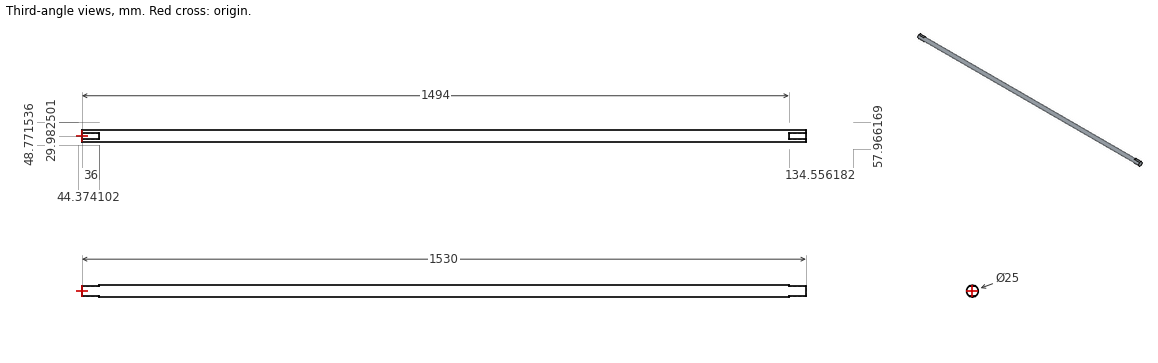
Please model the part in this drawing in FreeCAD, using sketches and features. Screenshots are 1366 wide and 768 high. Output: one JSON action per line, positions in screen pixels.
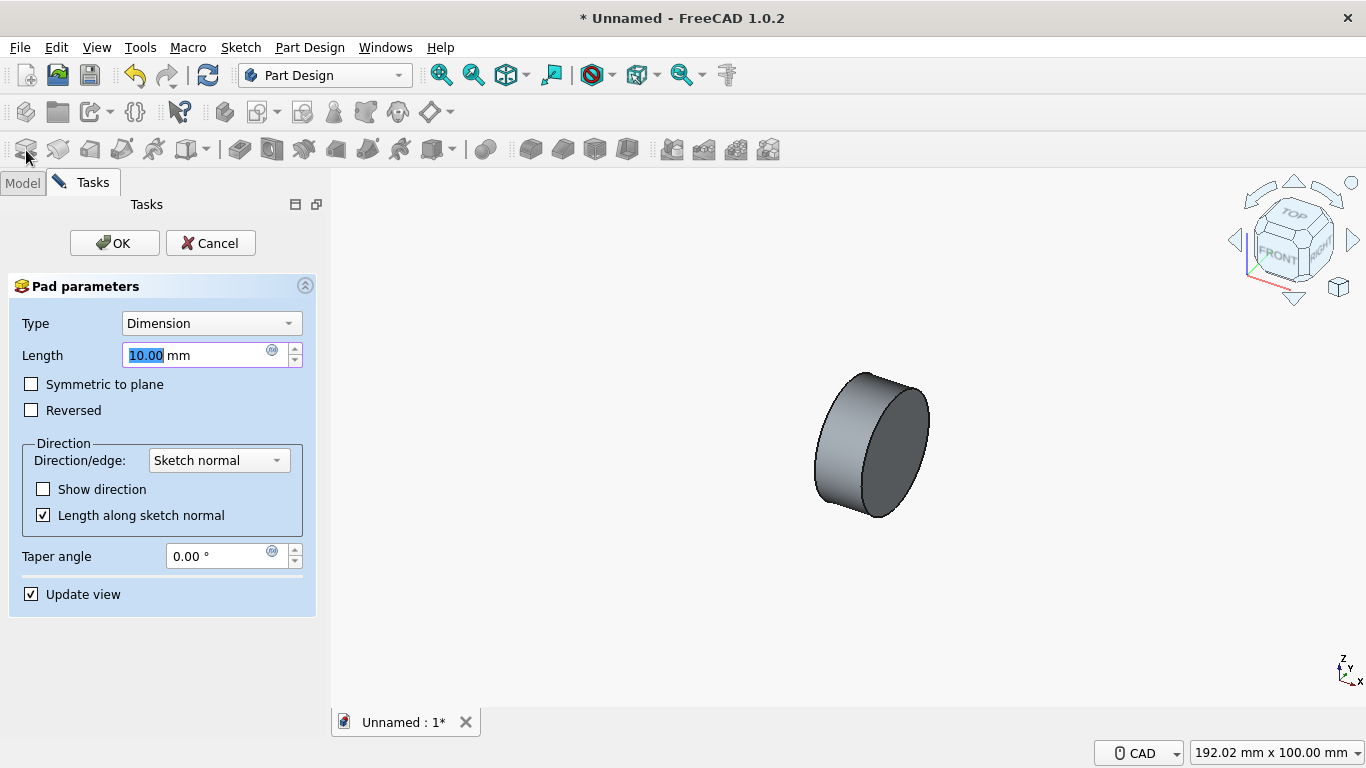
{"action": "type", "text": "1530"}
{"action": "key", "text": "Tab"}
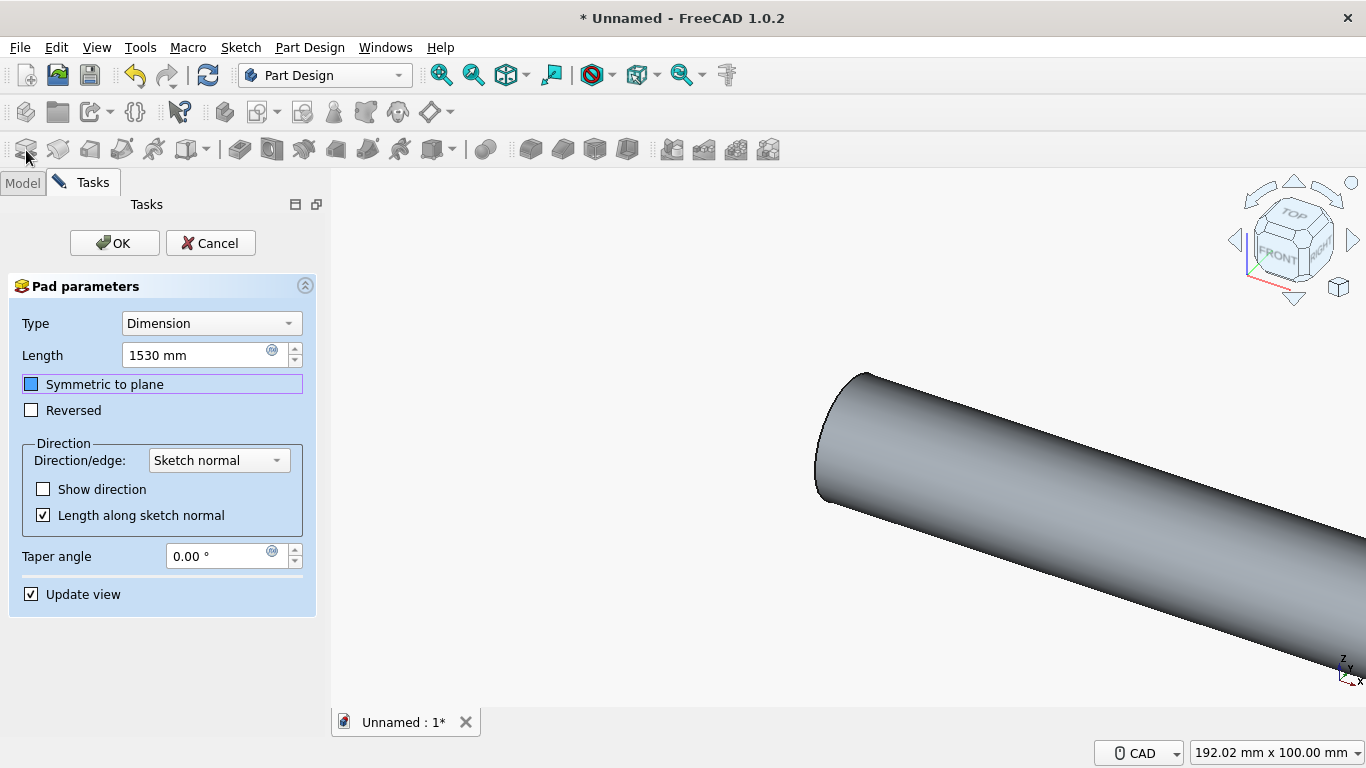
{"action": "left_click", "coordinate": [115, 243]}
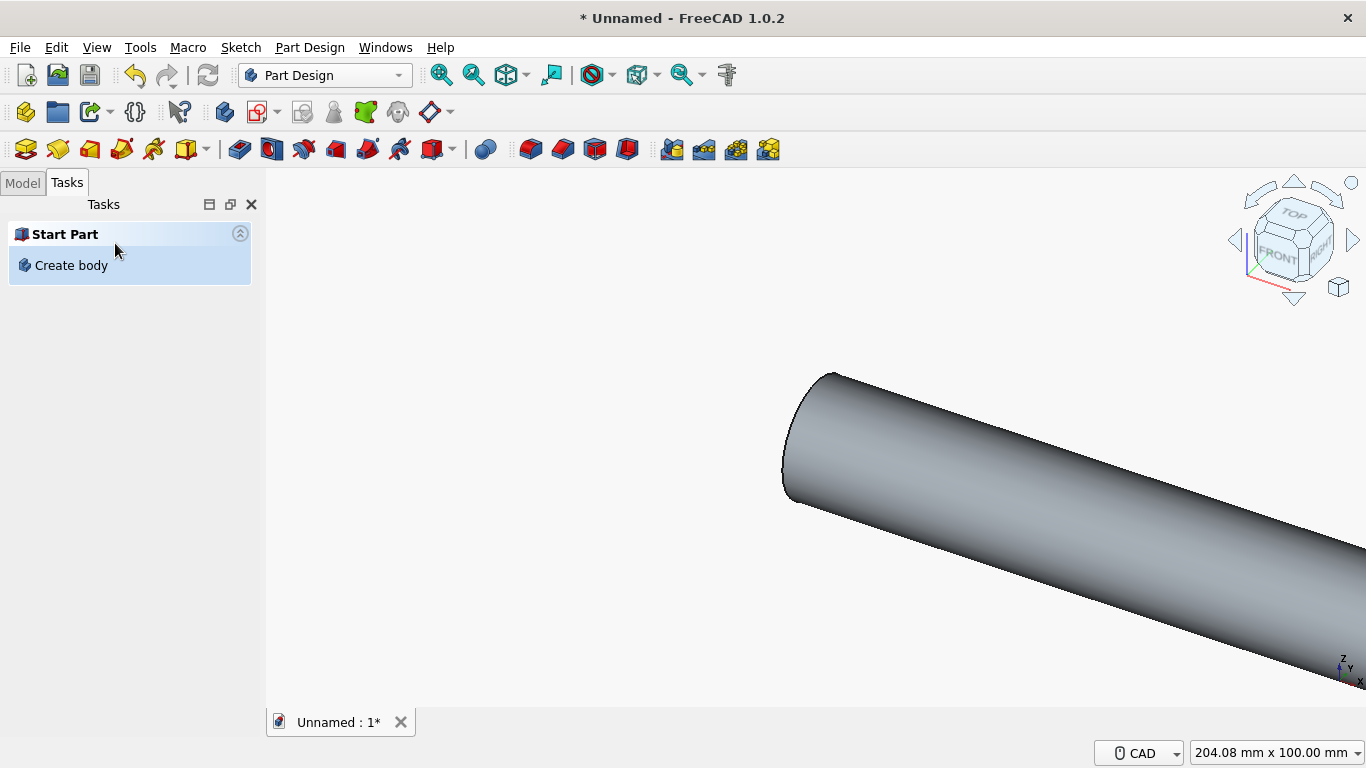
{"action": "left_click", "coordinate": [442, 76]}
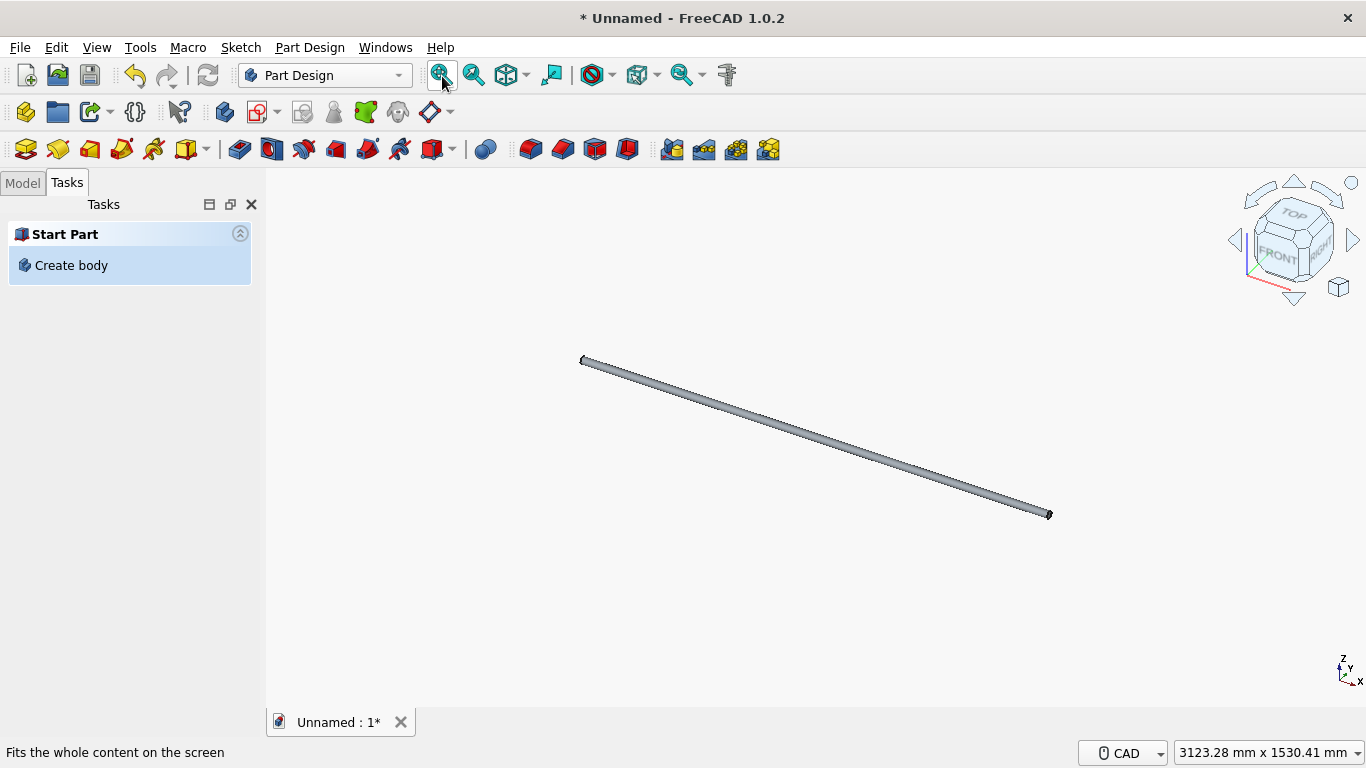
{"action": "left_click", "coordinate": [23, 182]}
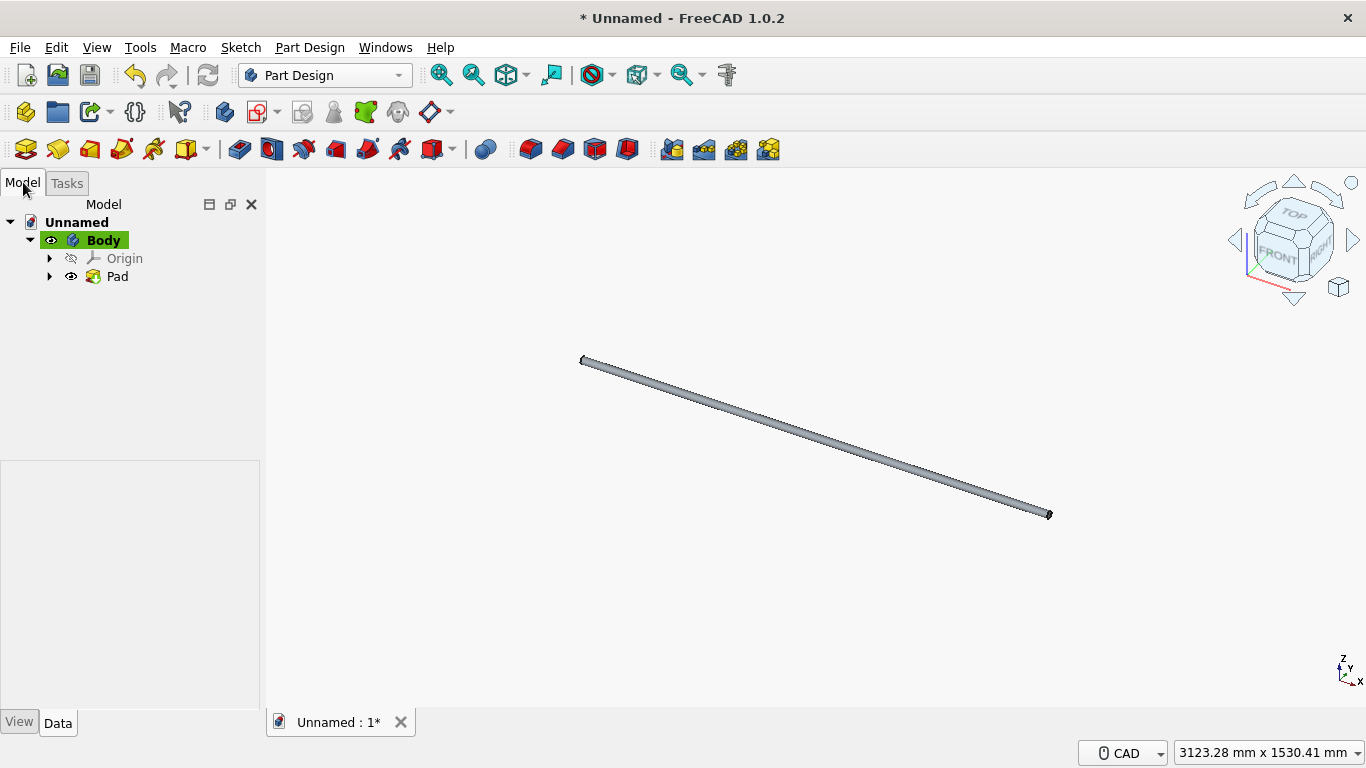
{"action": "left_click", "coordinate": [50, 258]}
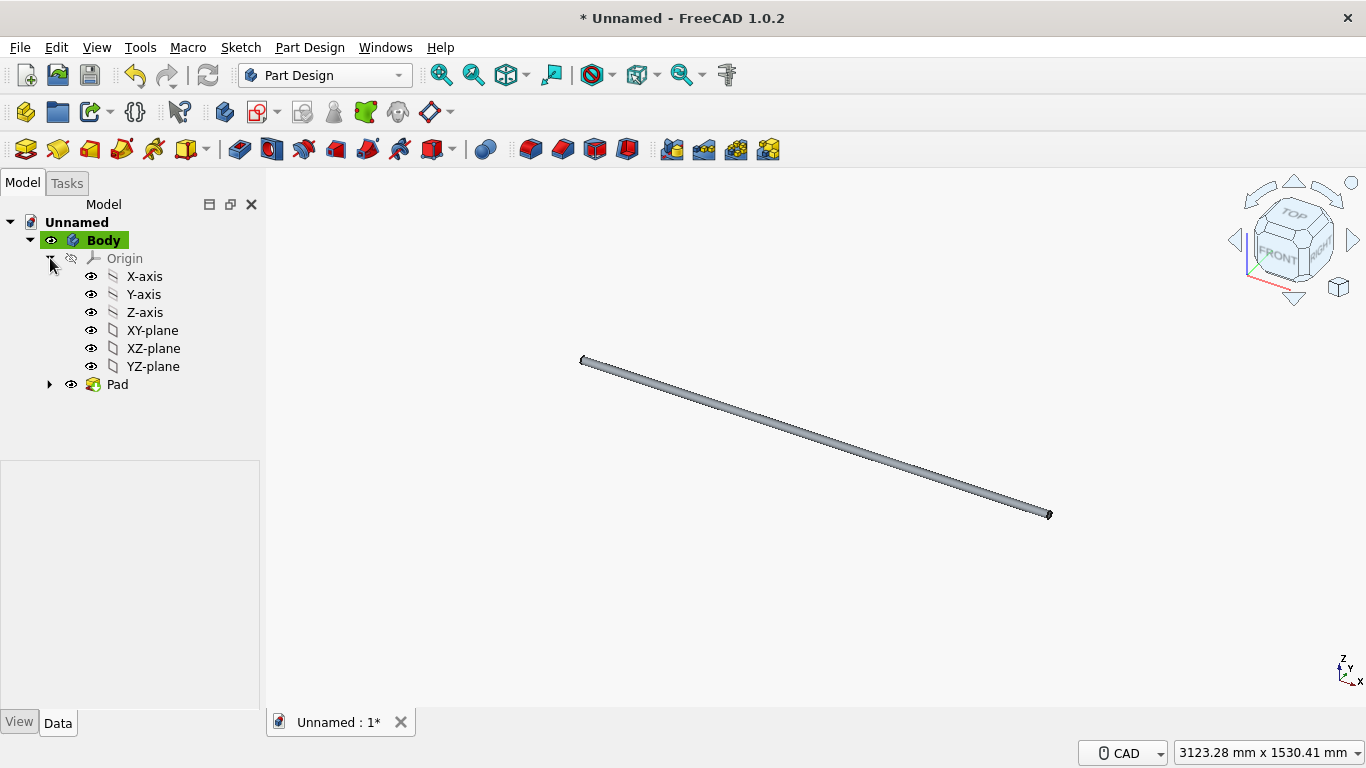
{"action": "left_click", "coordinate": [136, 330]}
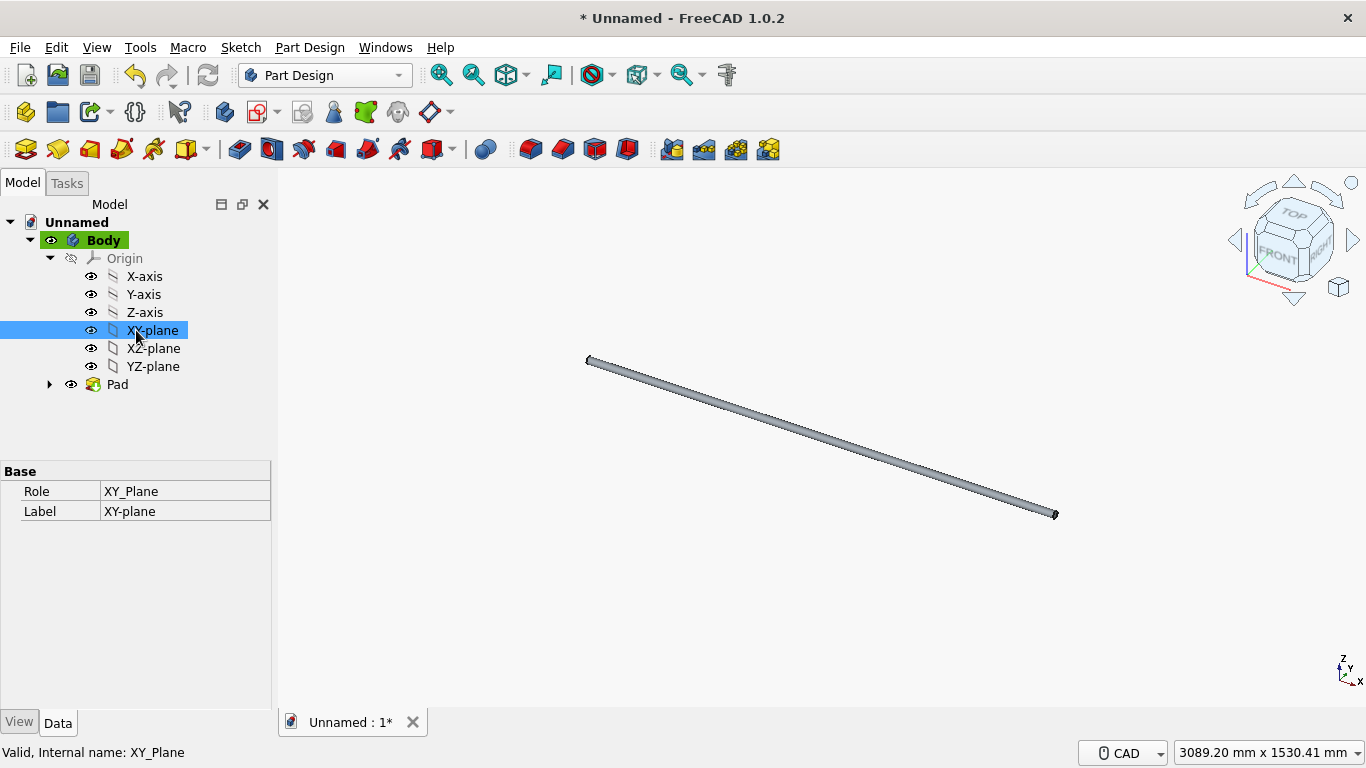
{"action": "left_click", "coordinate": [430, 112]}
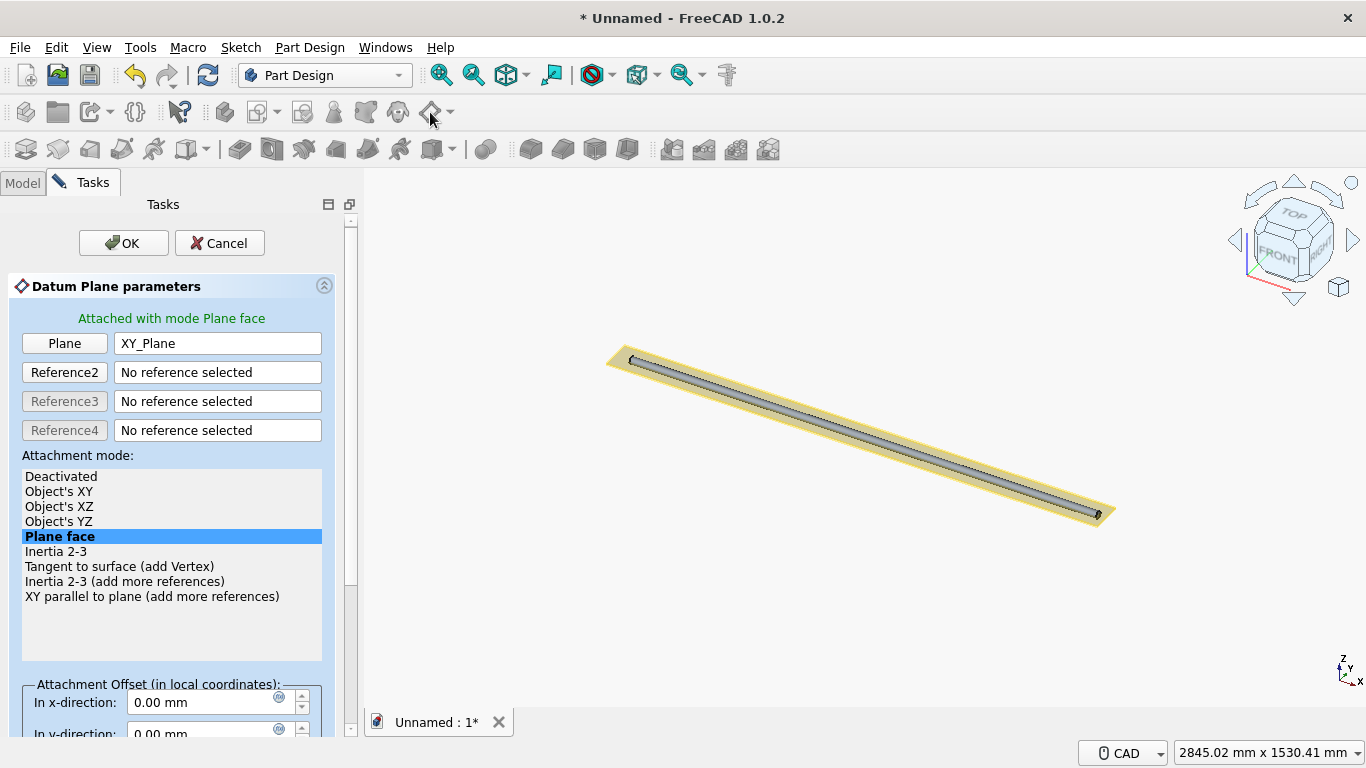
{"action": "scroll", "coordinate": [351, 475], "scroll_direction": "down", "scroll_amount": 2}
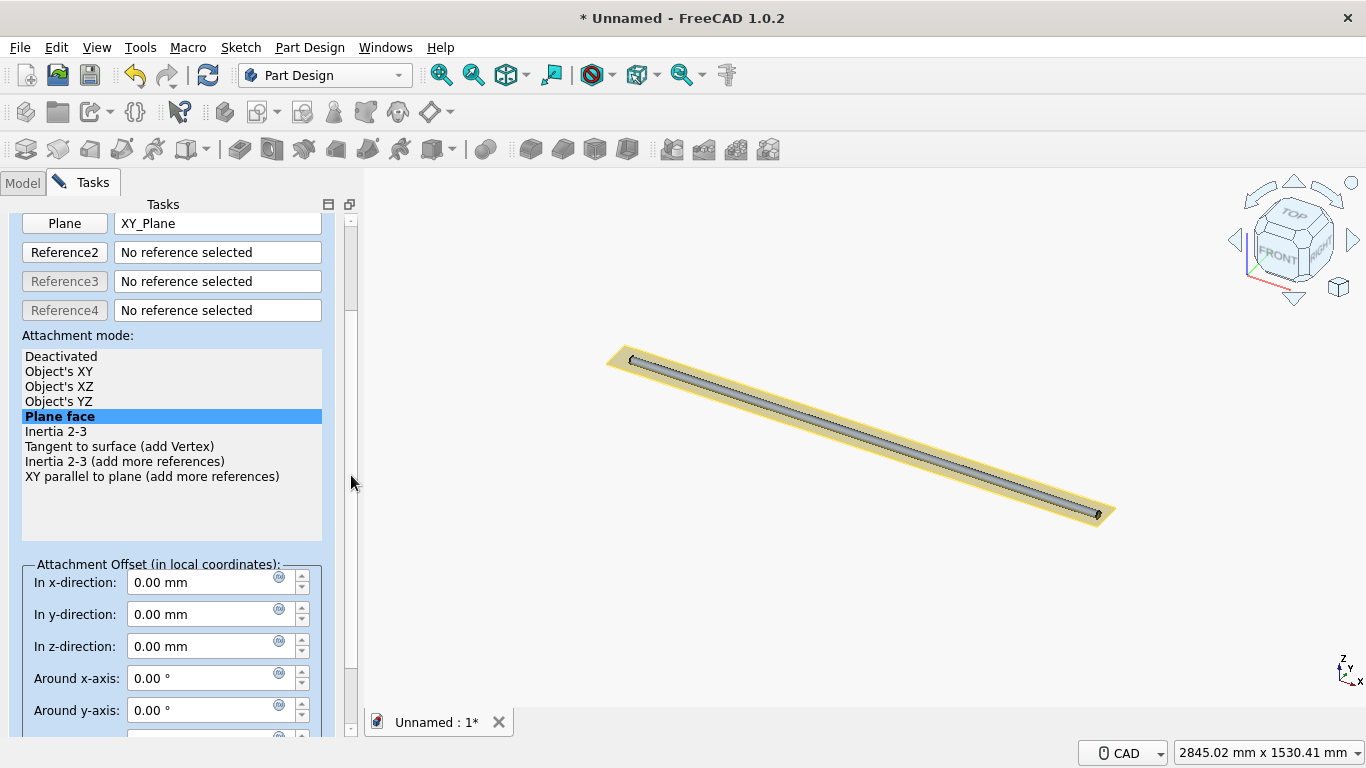
{"action": "triple_click", "coordinate": [210, 646]}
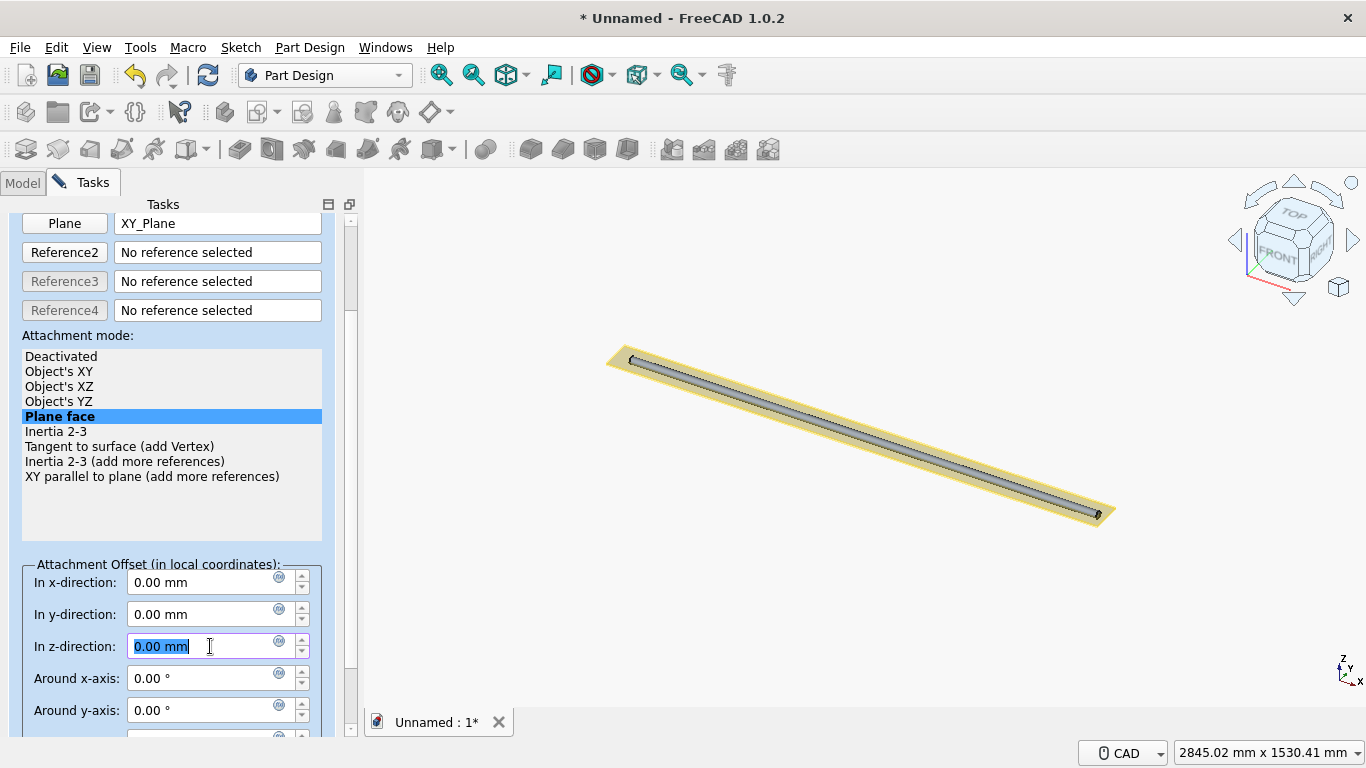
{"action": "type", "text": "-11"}
{"action": "key", "text": "Tab"}